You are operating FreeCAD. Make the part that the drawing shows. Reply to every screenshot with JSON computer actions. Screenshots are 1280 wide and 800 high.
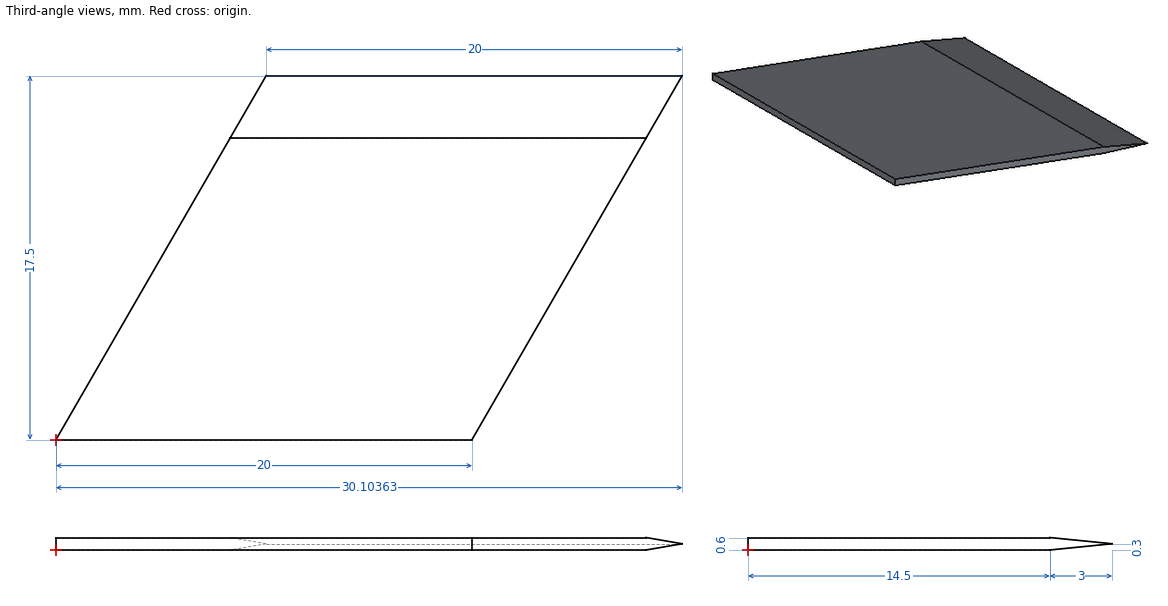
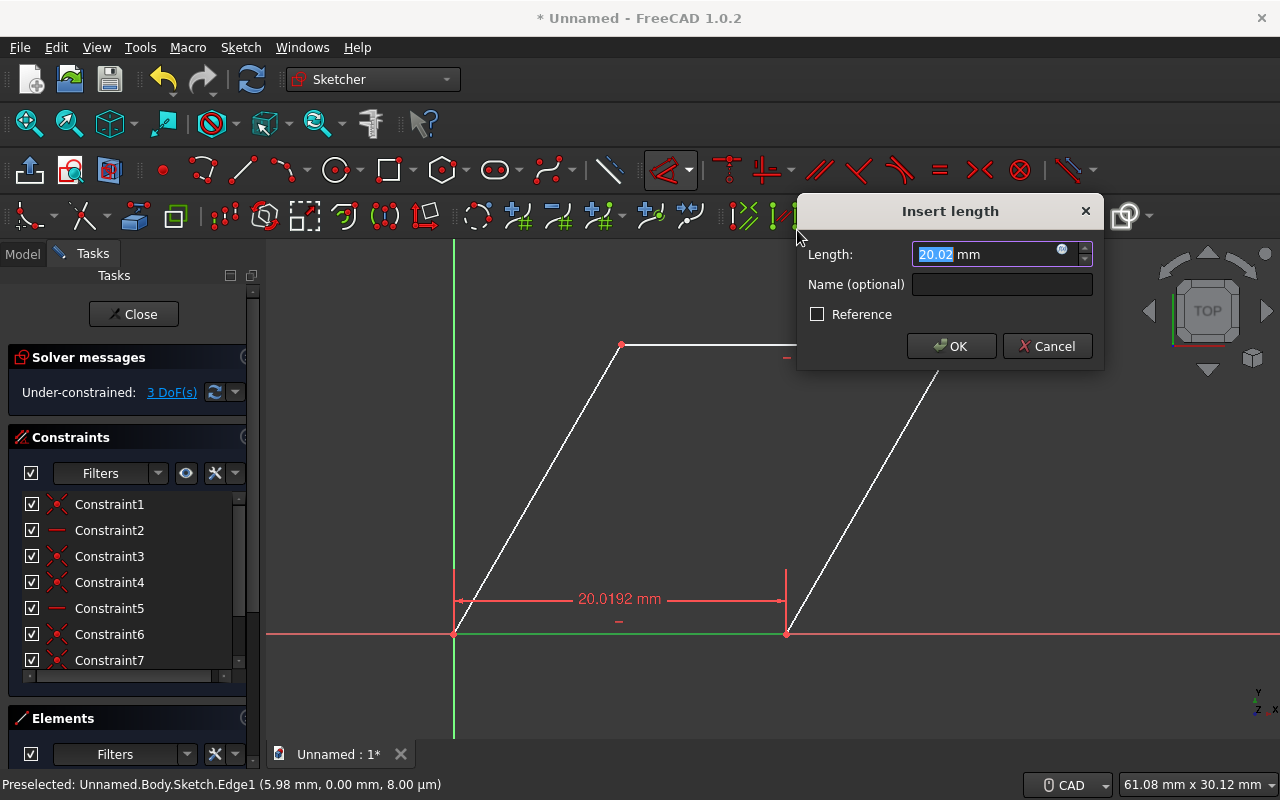
{"action": "type", "text": "20"}
{"action": "key", "text": "Return"}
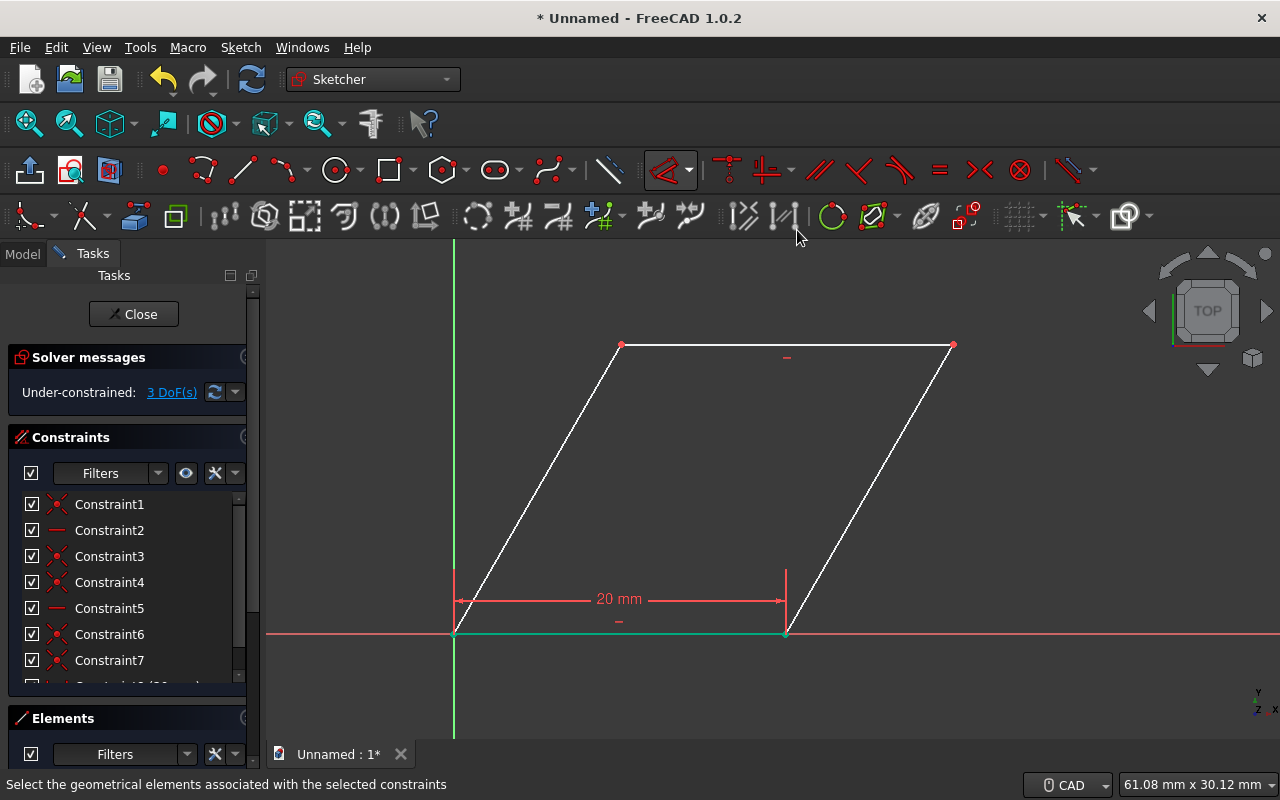
{"action": "left_click", "coordinate": [853, 345]}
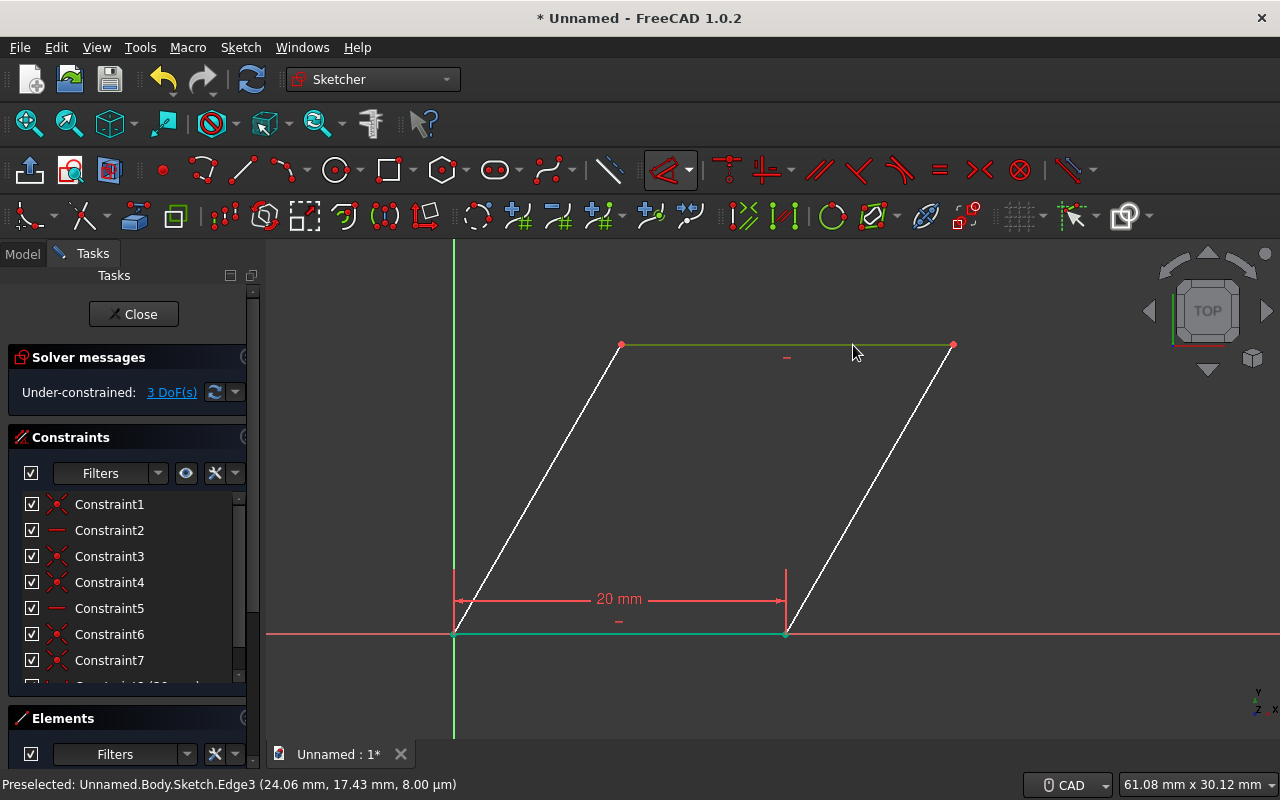
{"action": "key", "text": "l"}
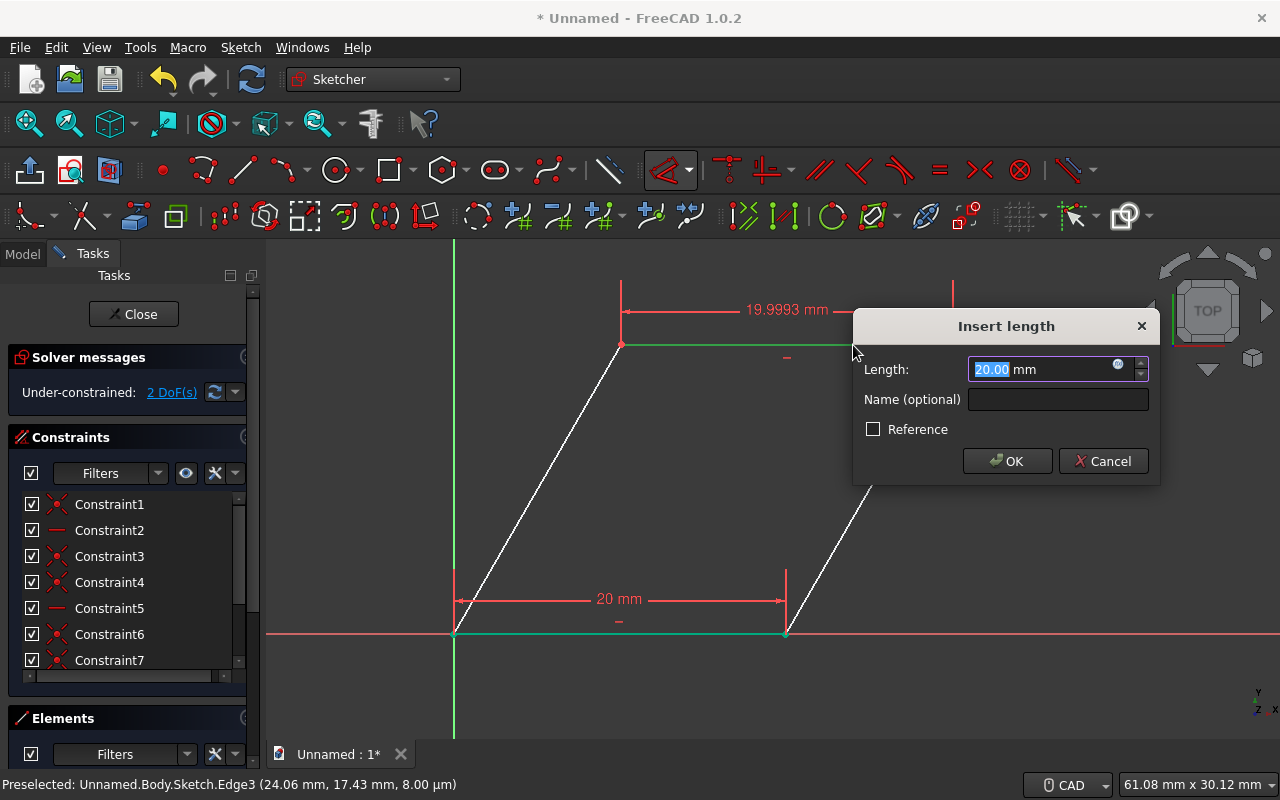
{"action": "type", "text": "20"}
{"action": "key", "text": "Return"}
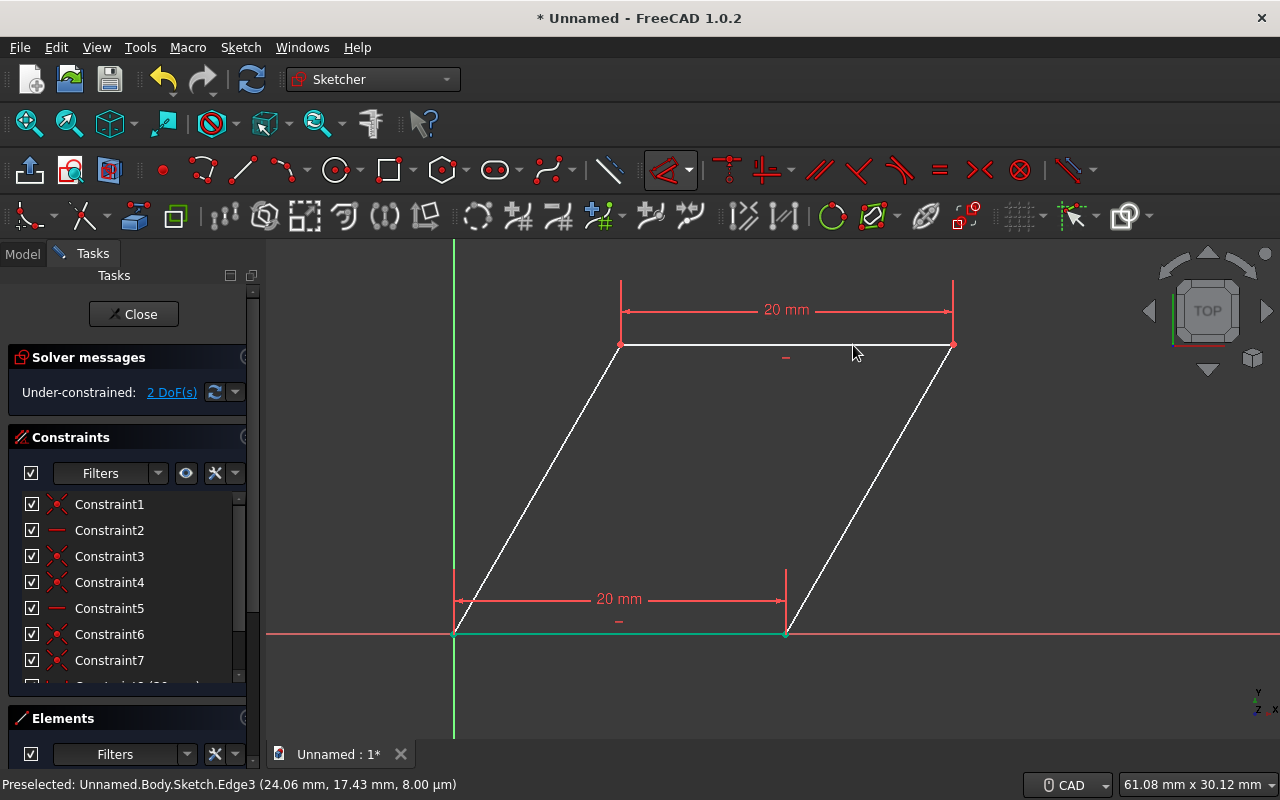
{"action": "left_click", "coordinate": [953, 345]}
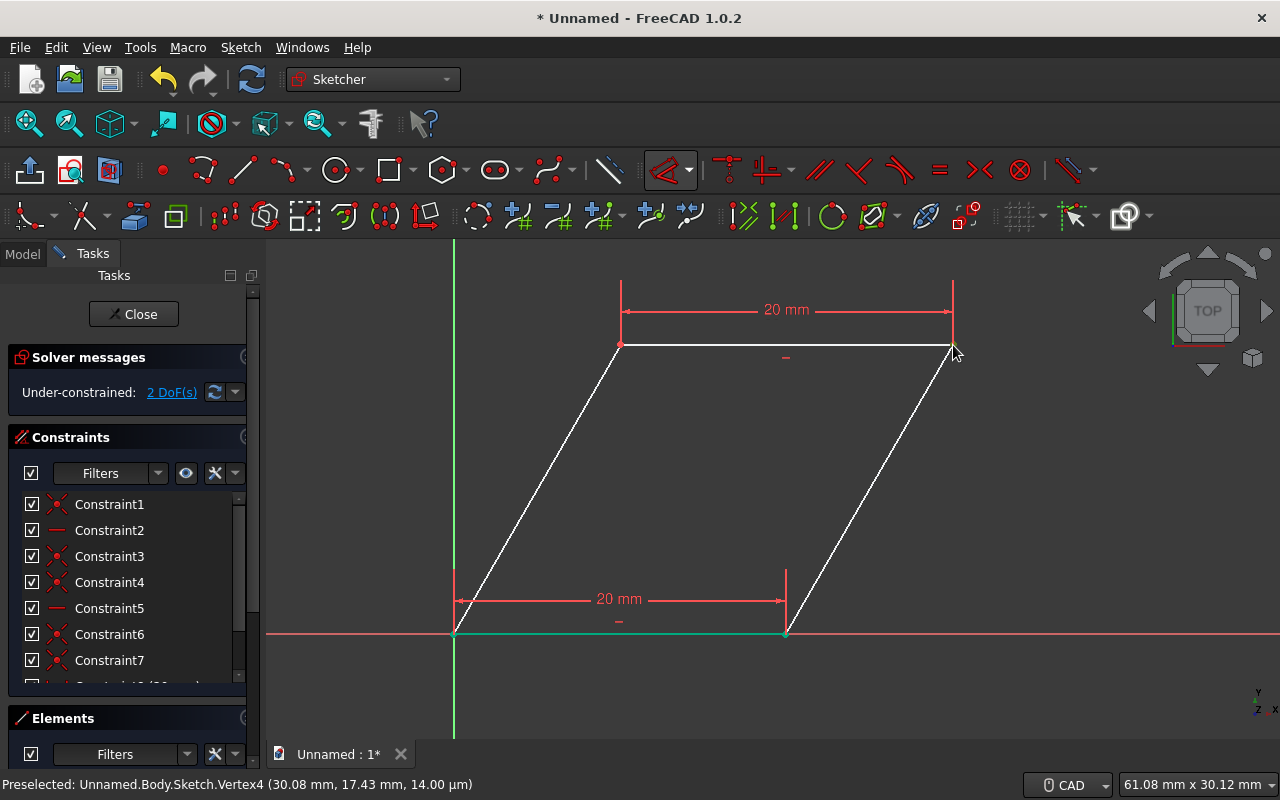
{"action": "key", "text": "i"}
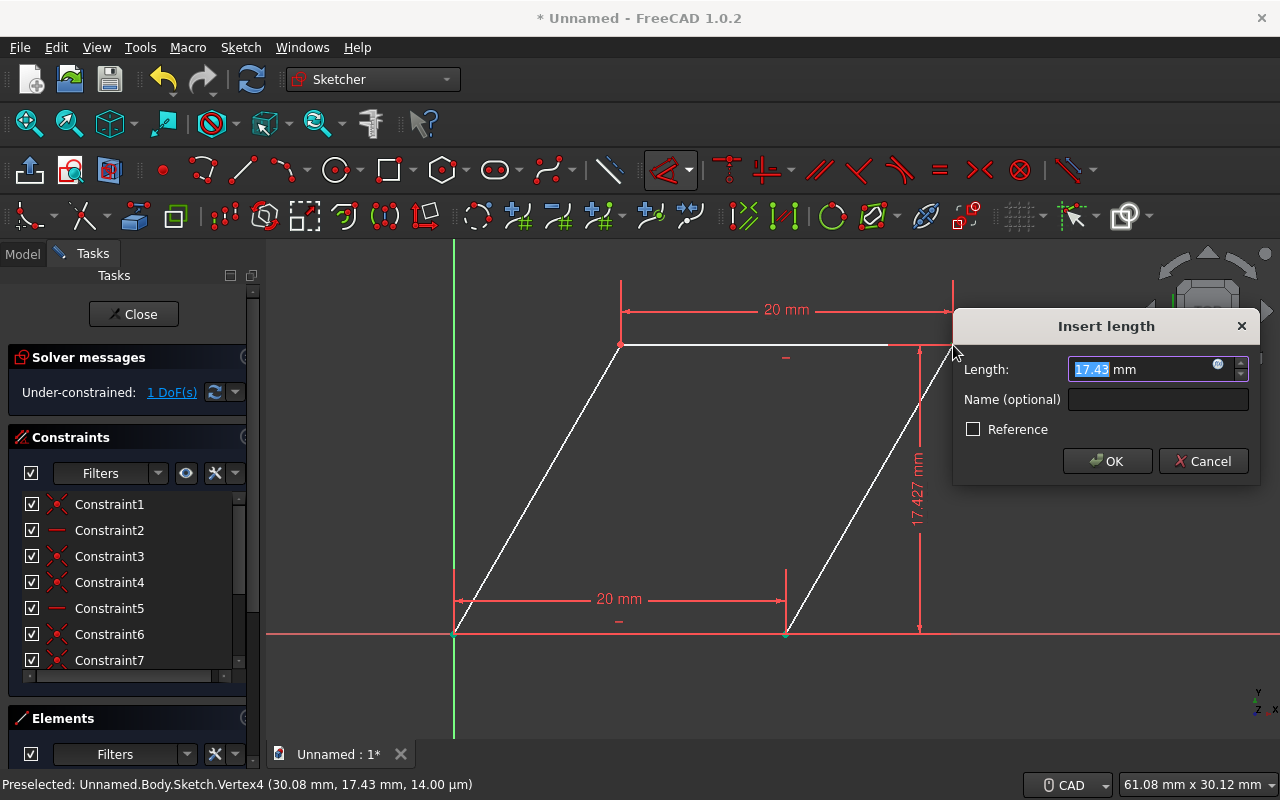
{"action": "type", "text": "17.5"}
{"action": "key", "text": "Return"}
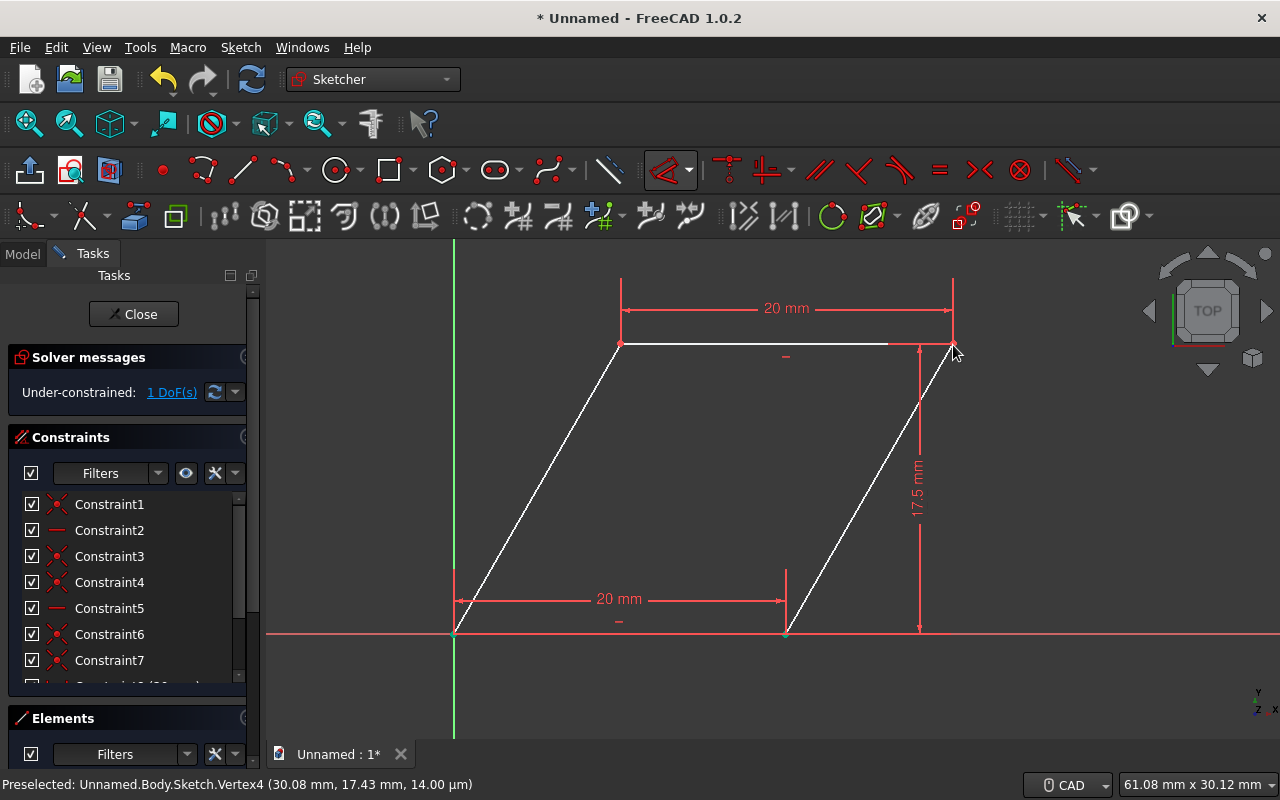
{"action": "left_click", "coordinate": [953, 344]}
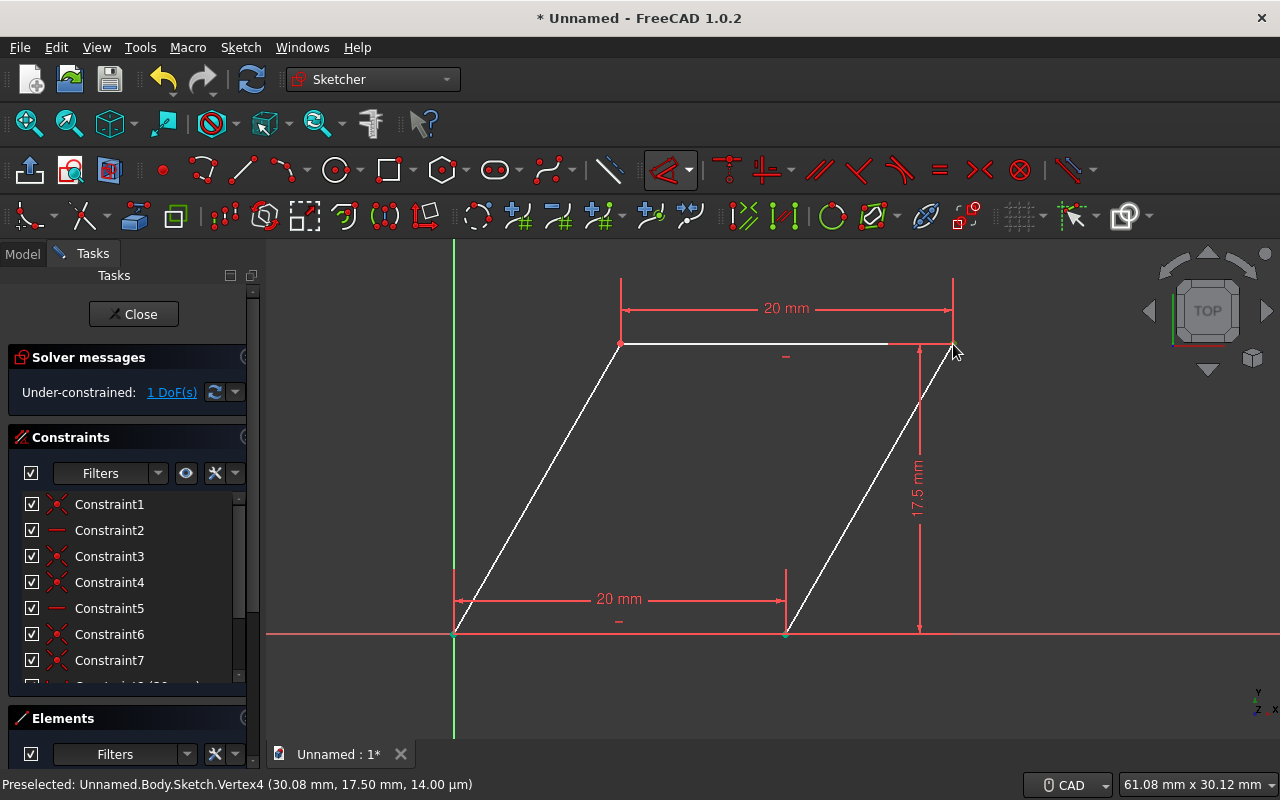
{"action": "left_click", "coordinate": [692, 170]}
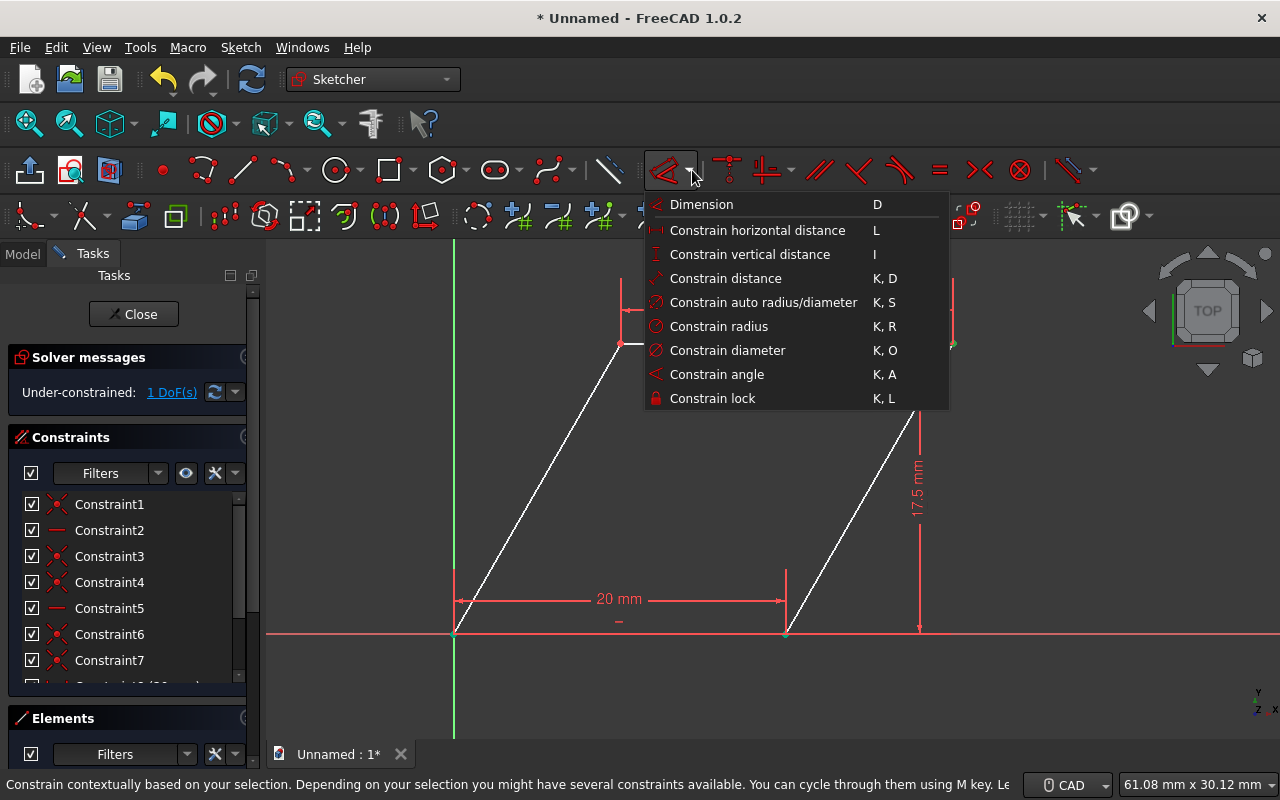
{"action": "left_click", "coordinate": [797, 230]}